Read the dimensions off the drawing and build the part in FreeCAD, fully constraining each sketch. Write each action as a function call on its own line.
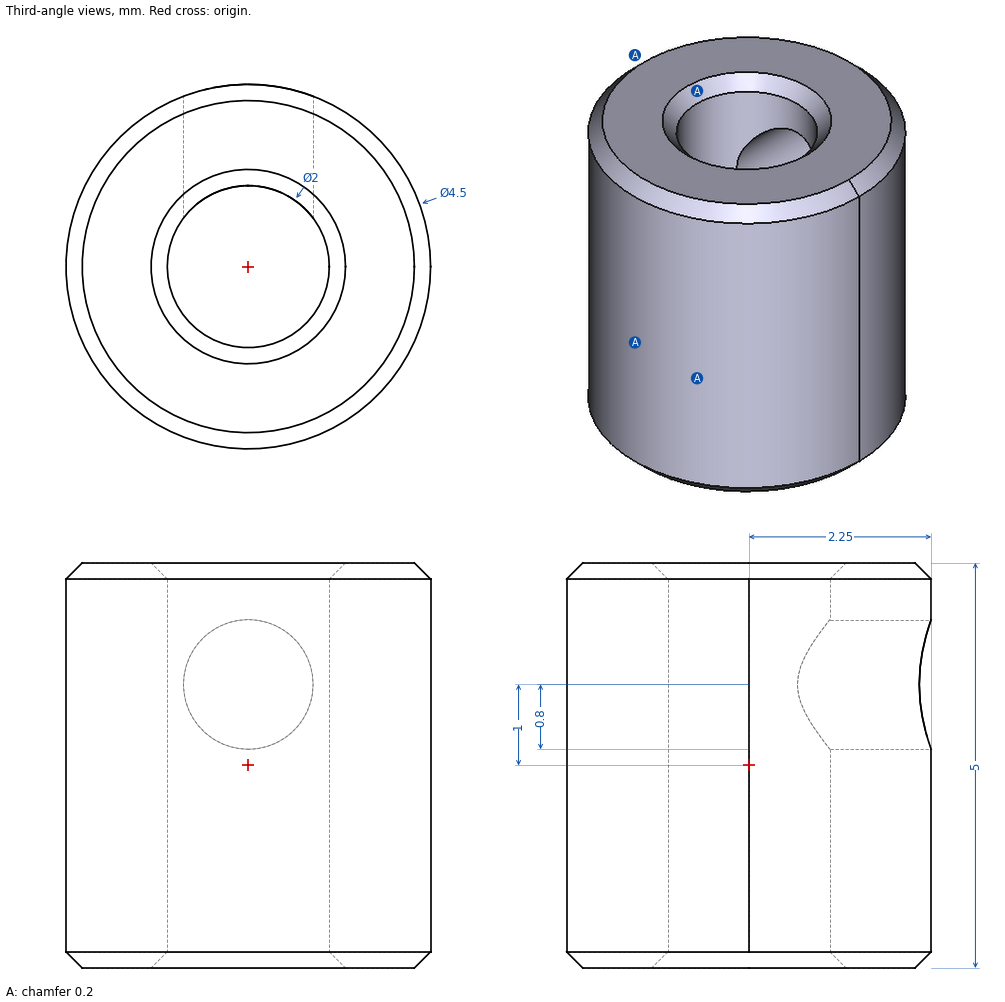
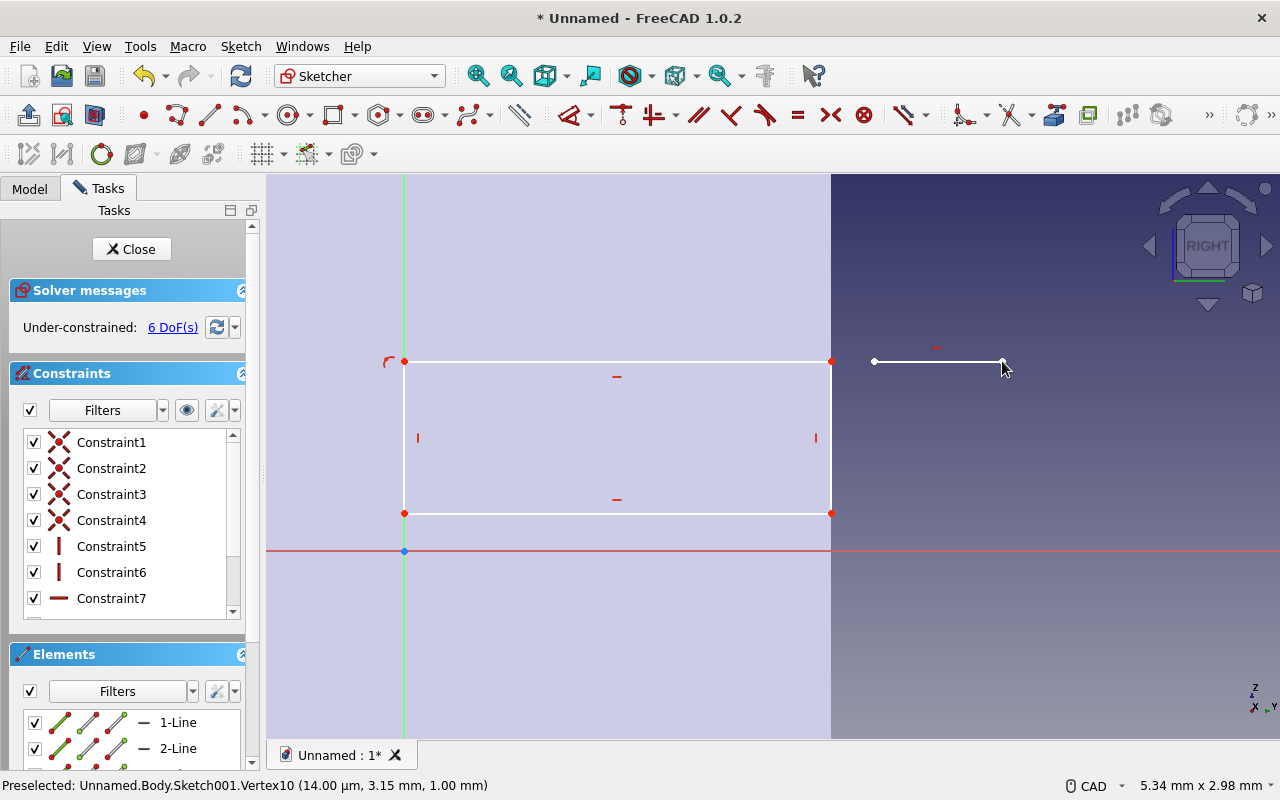
click(912, 362)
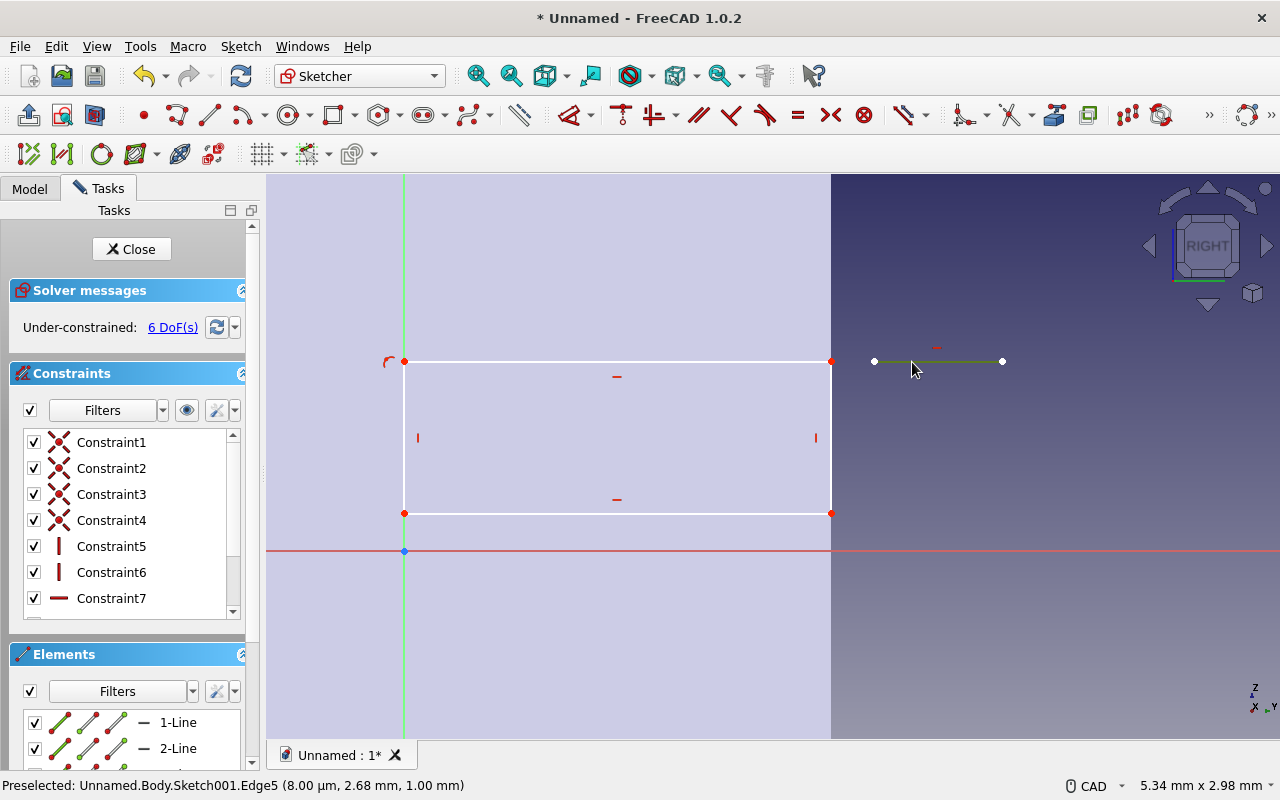
click(520, 116)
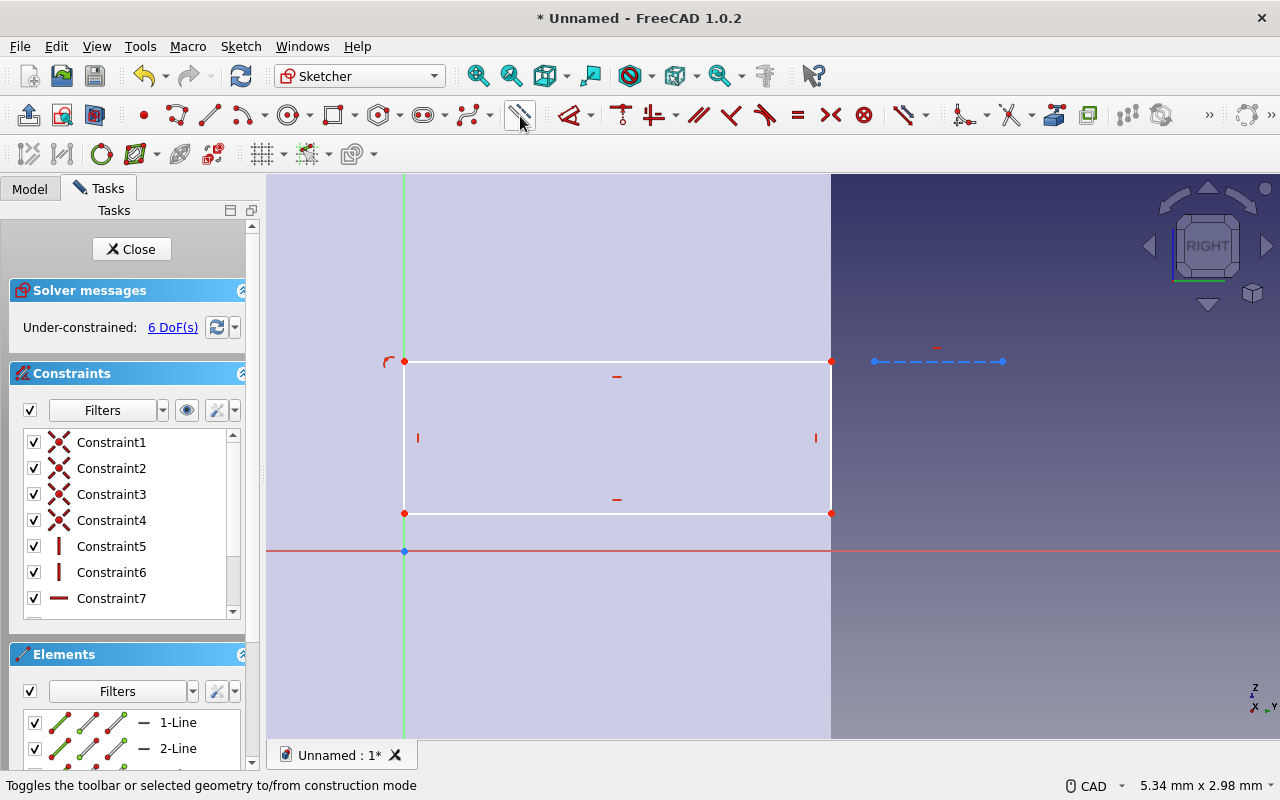
click(568, 116)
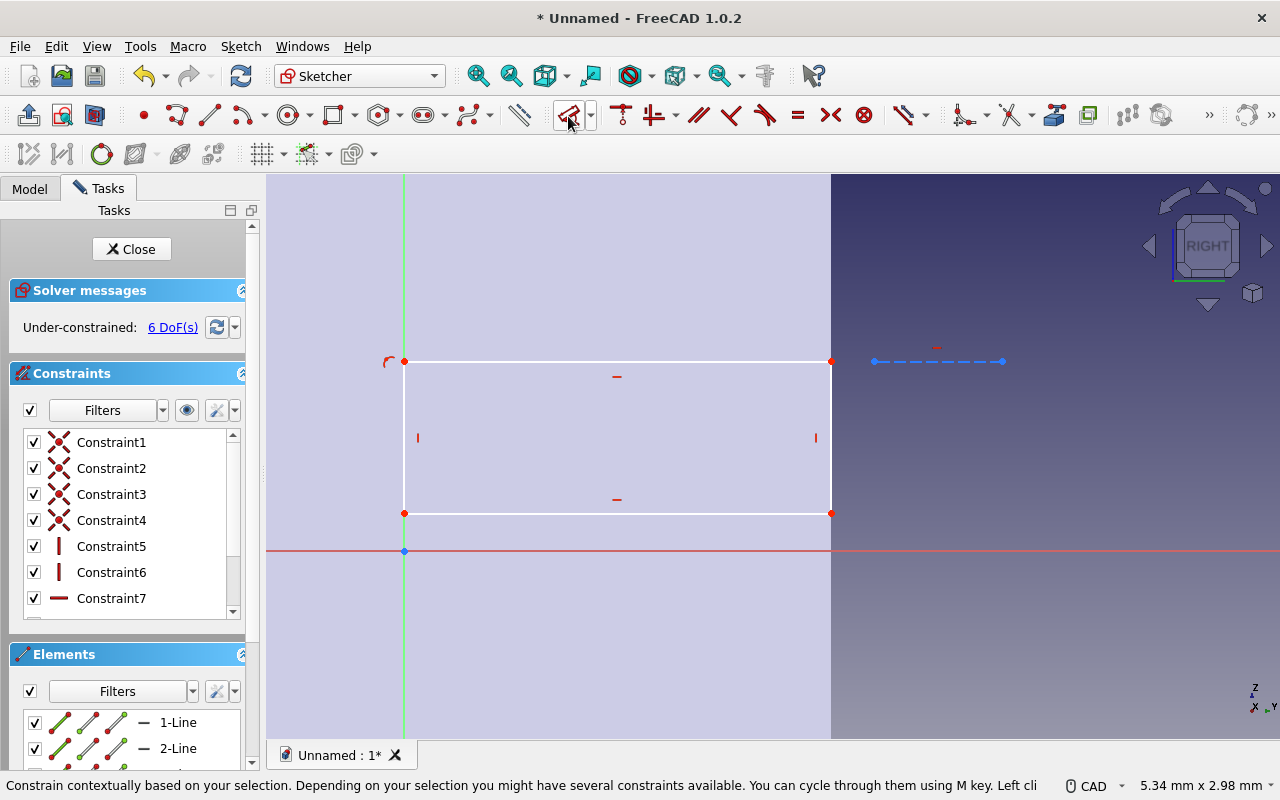
click(404, 362)
click(370, 457)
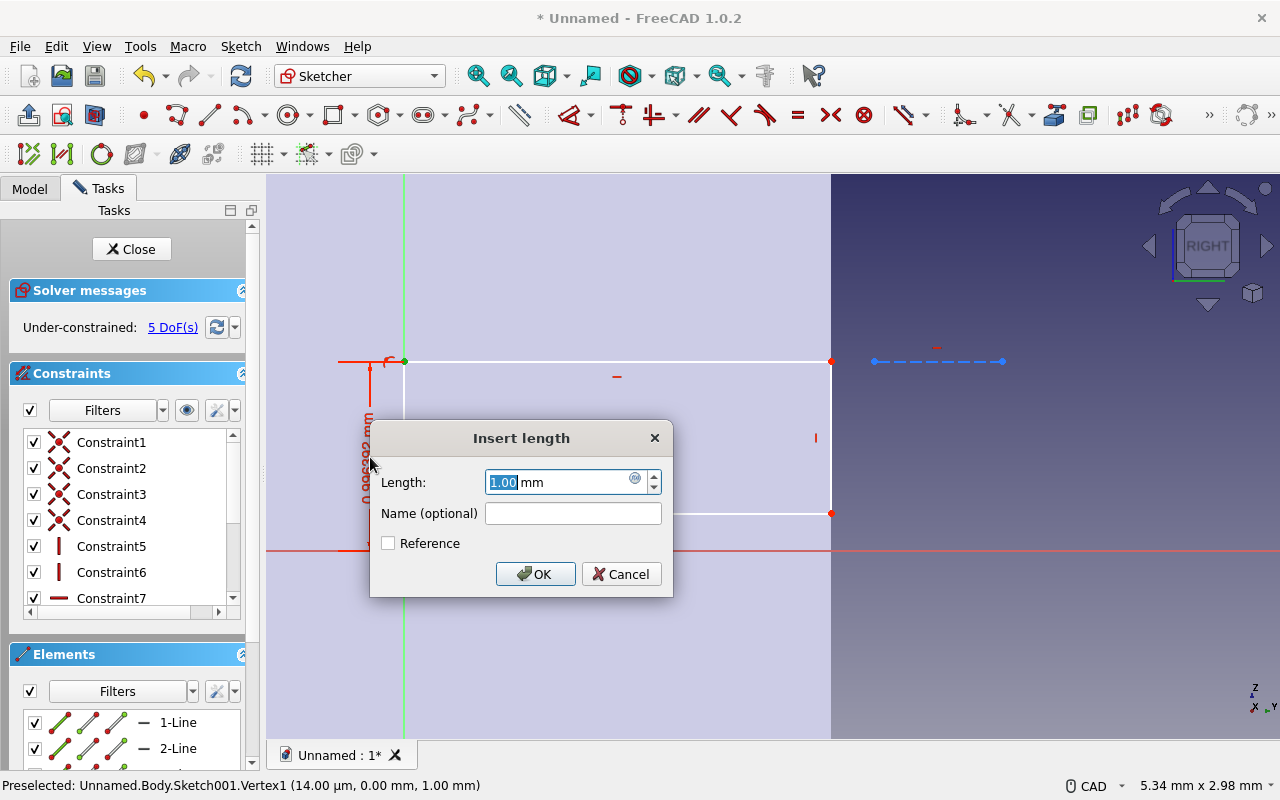
text(1)
key(Return)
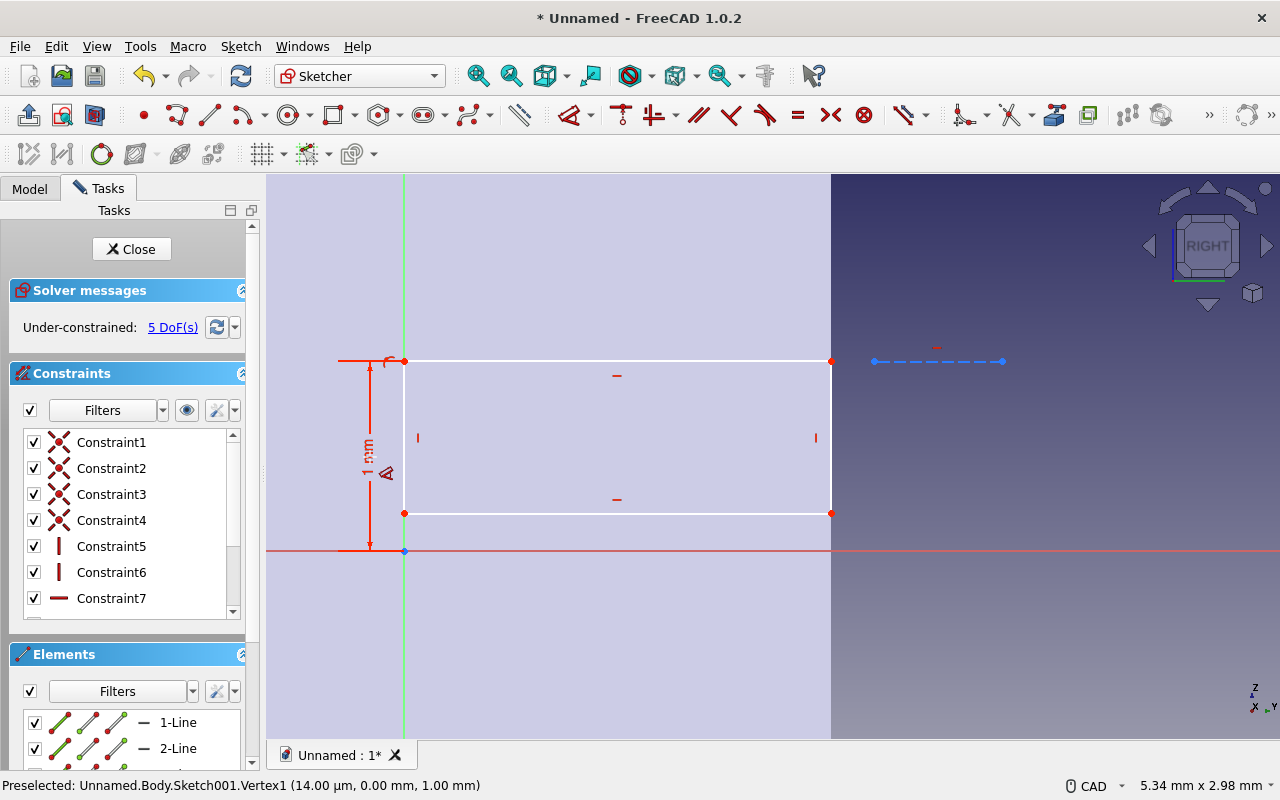
click(874, 362)
click(370, 413)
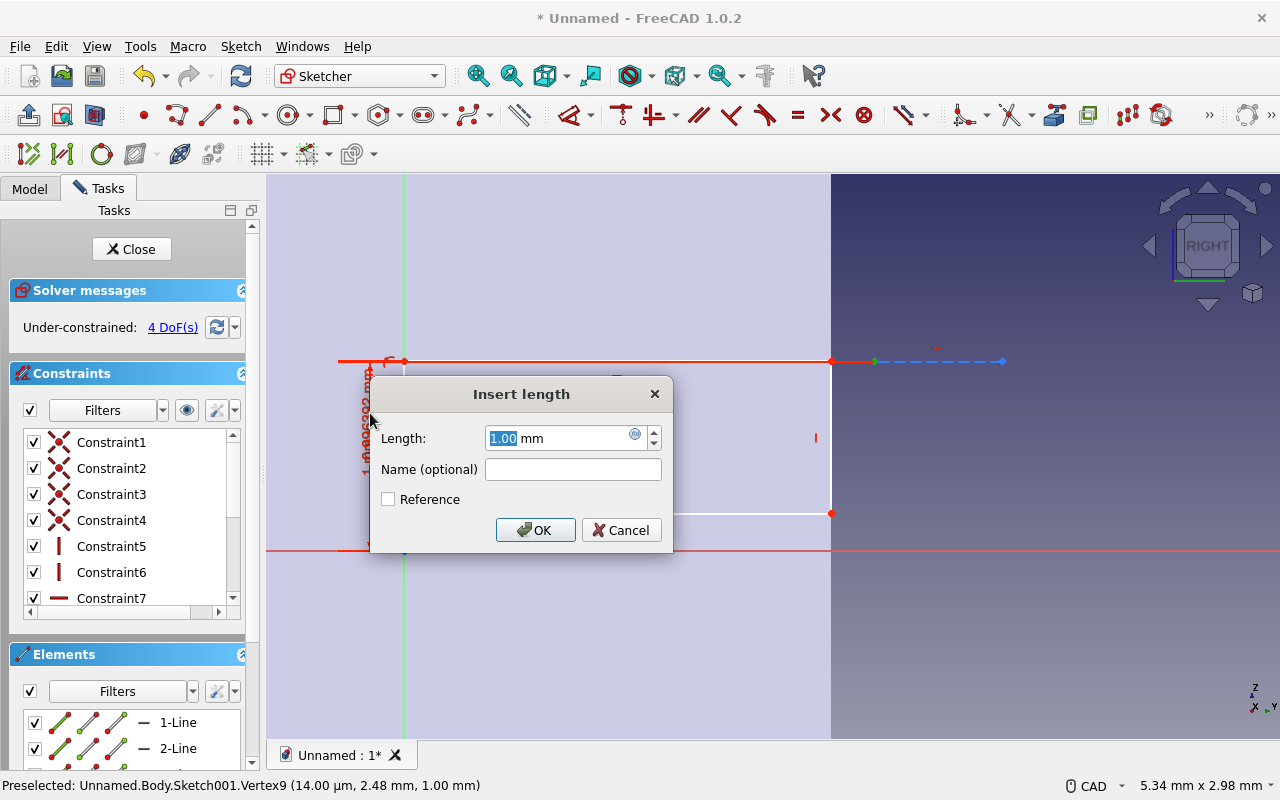
text(1)
key(Return)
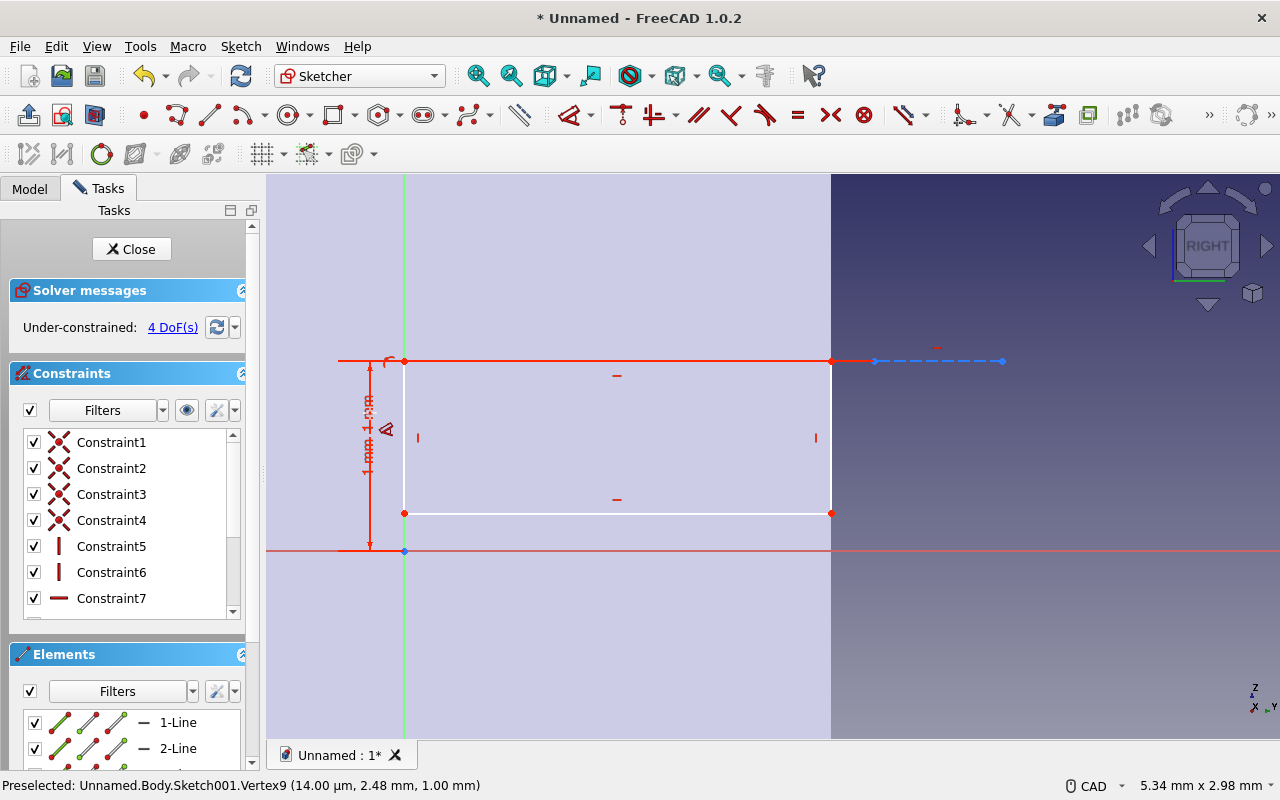
click(404, 407)
click(370, 384)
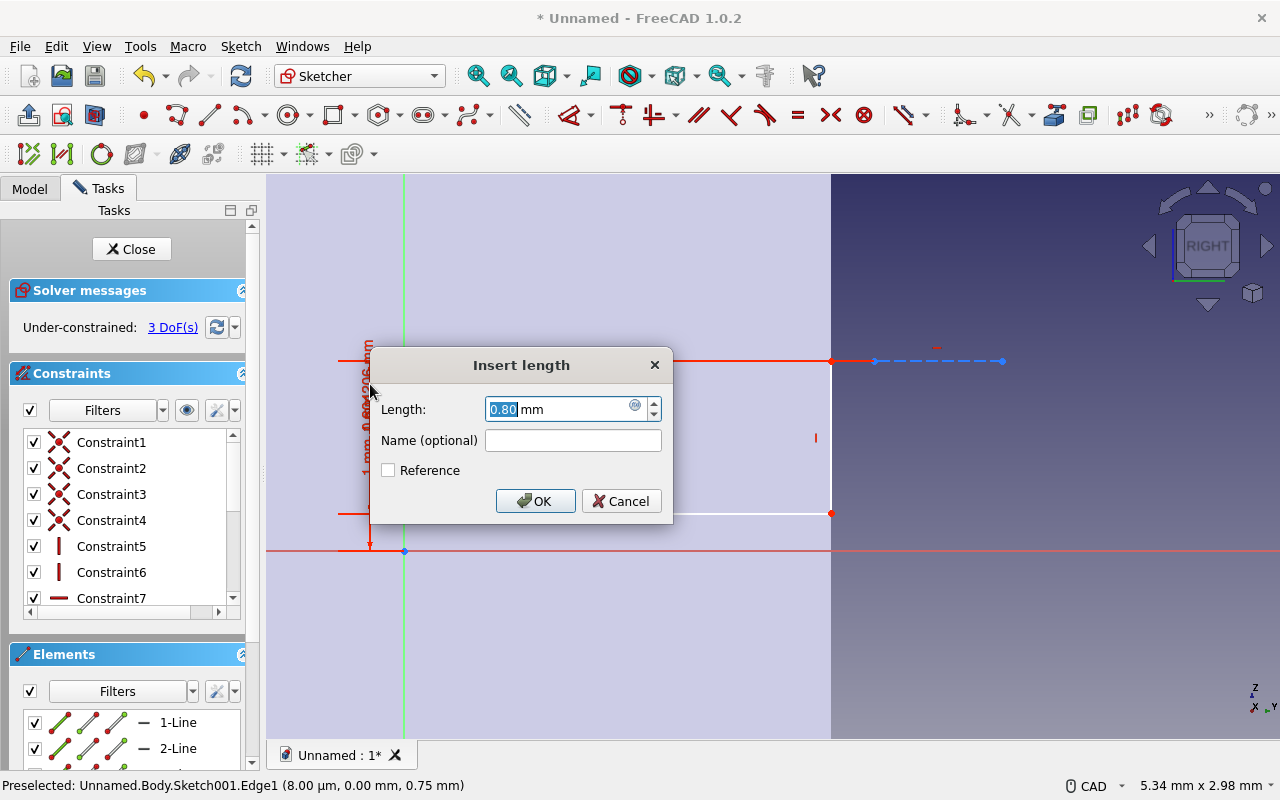
text(0.8)
key(Return)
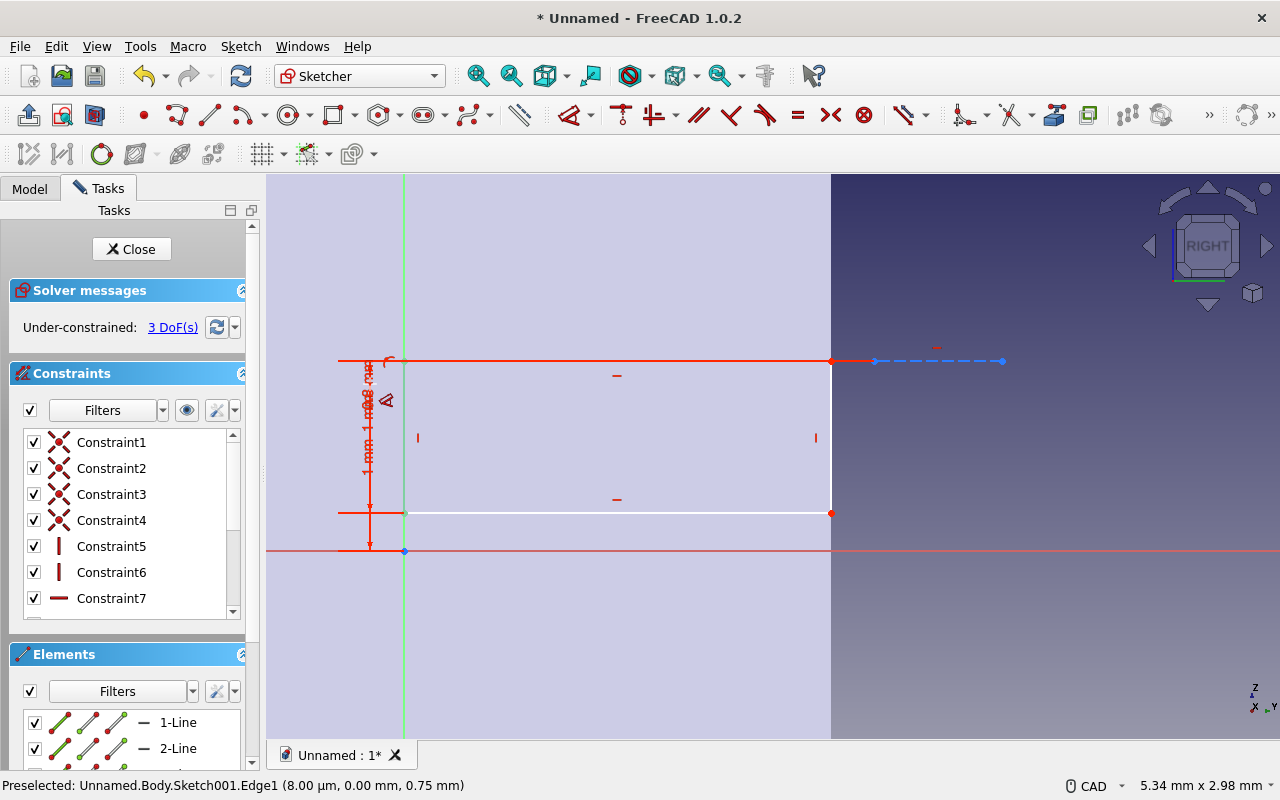
click(532, 513)
click(618, 479)